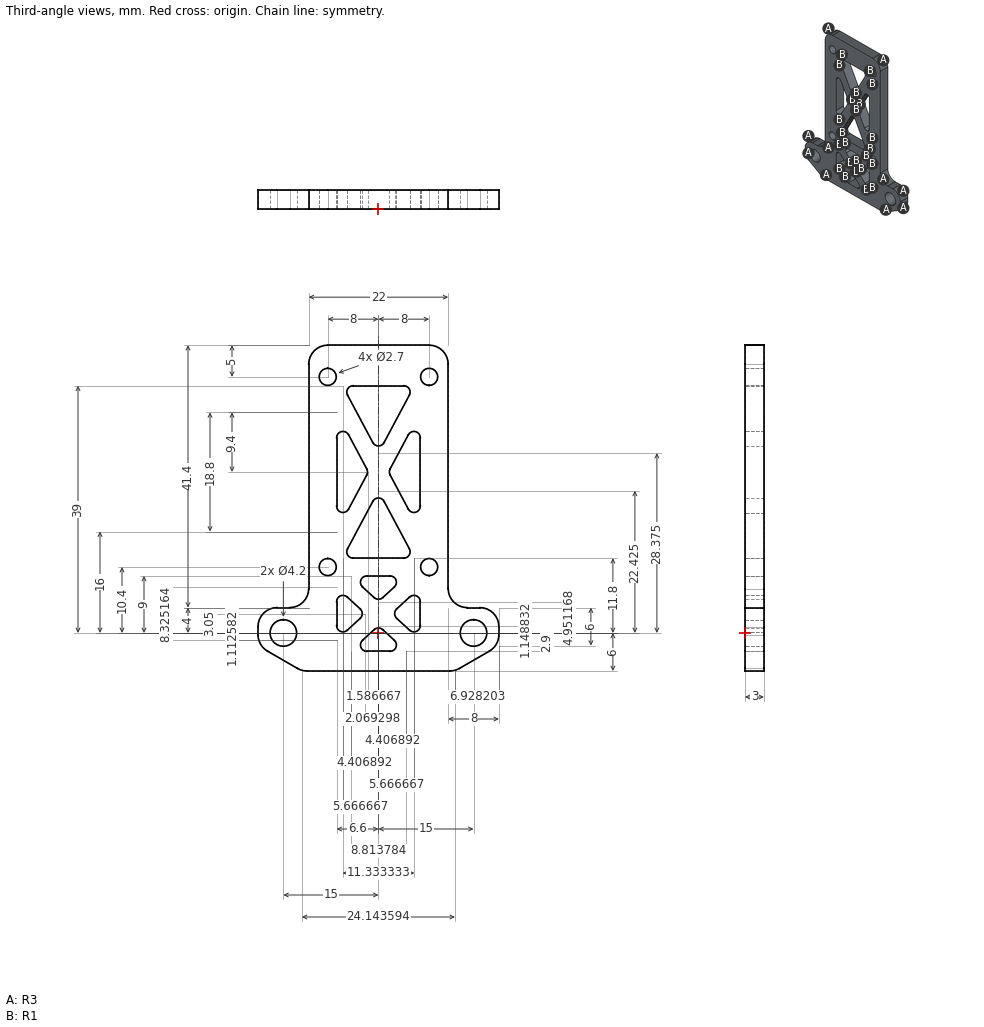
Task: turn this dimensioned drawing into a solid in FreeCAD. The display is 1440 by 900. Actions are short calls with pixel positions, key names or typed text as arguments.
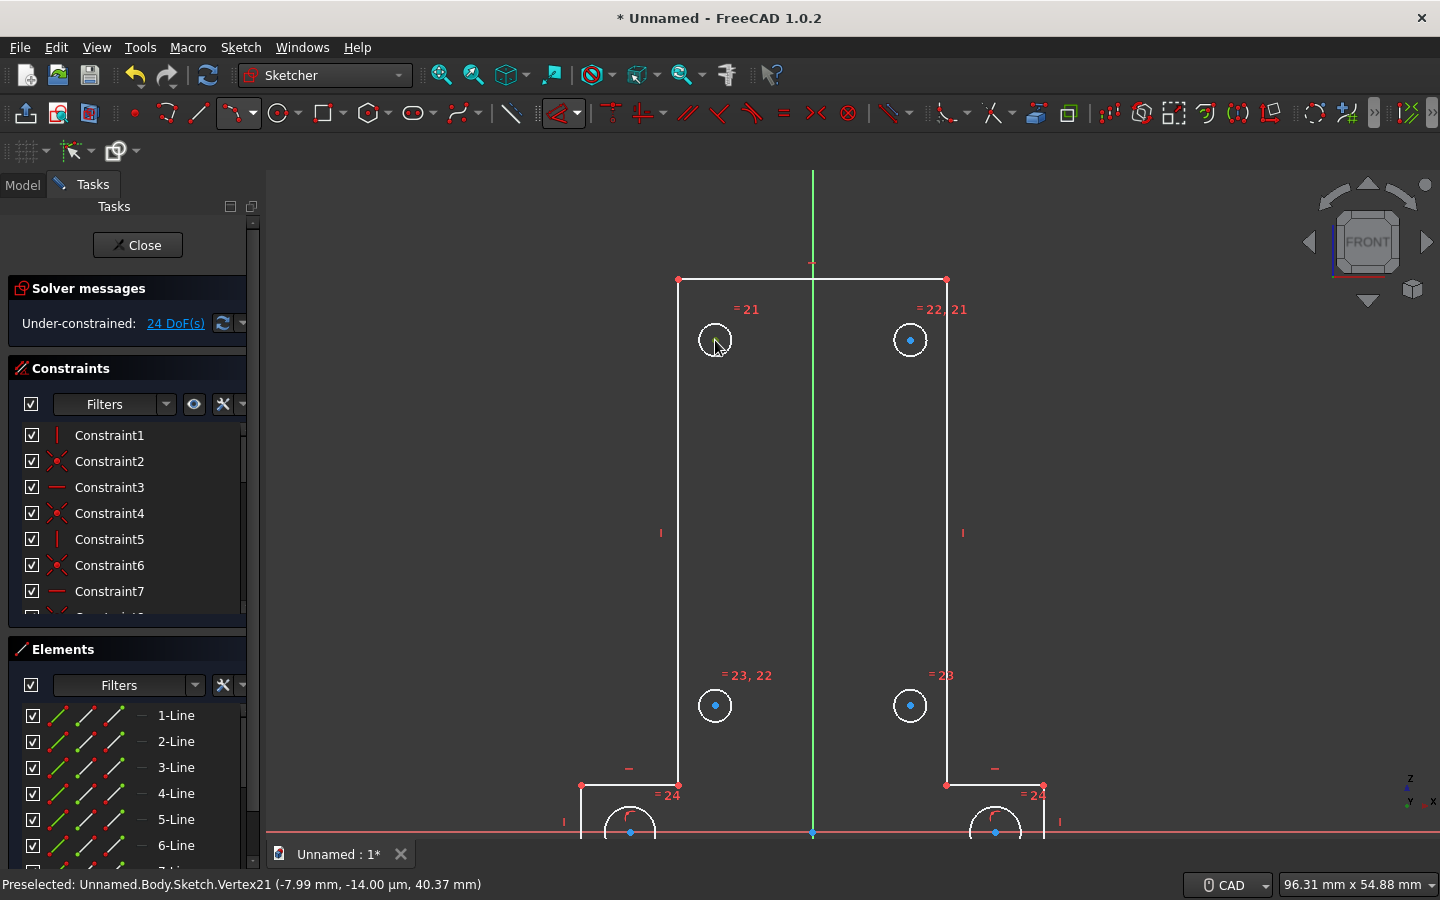
click(910, 340)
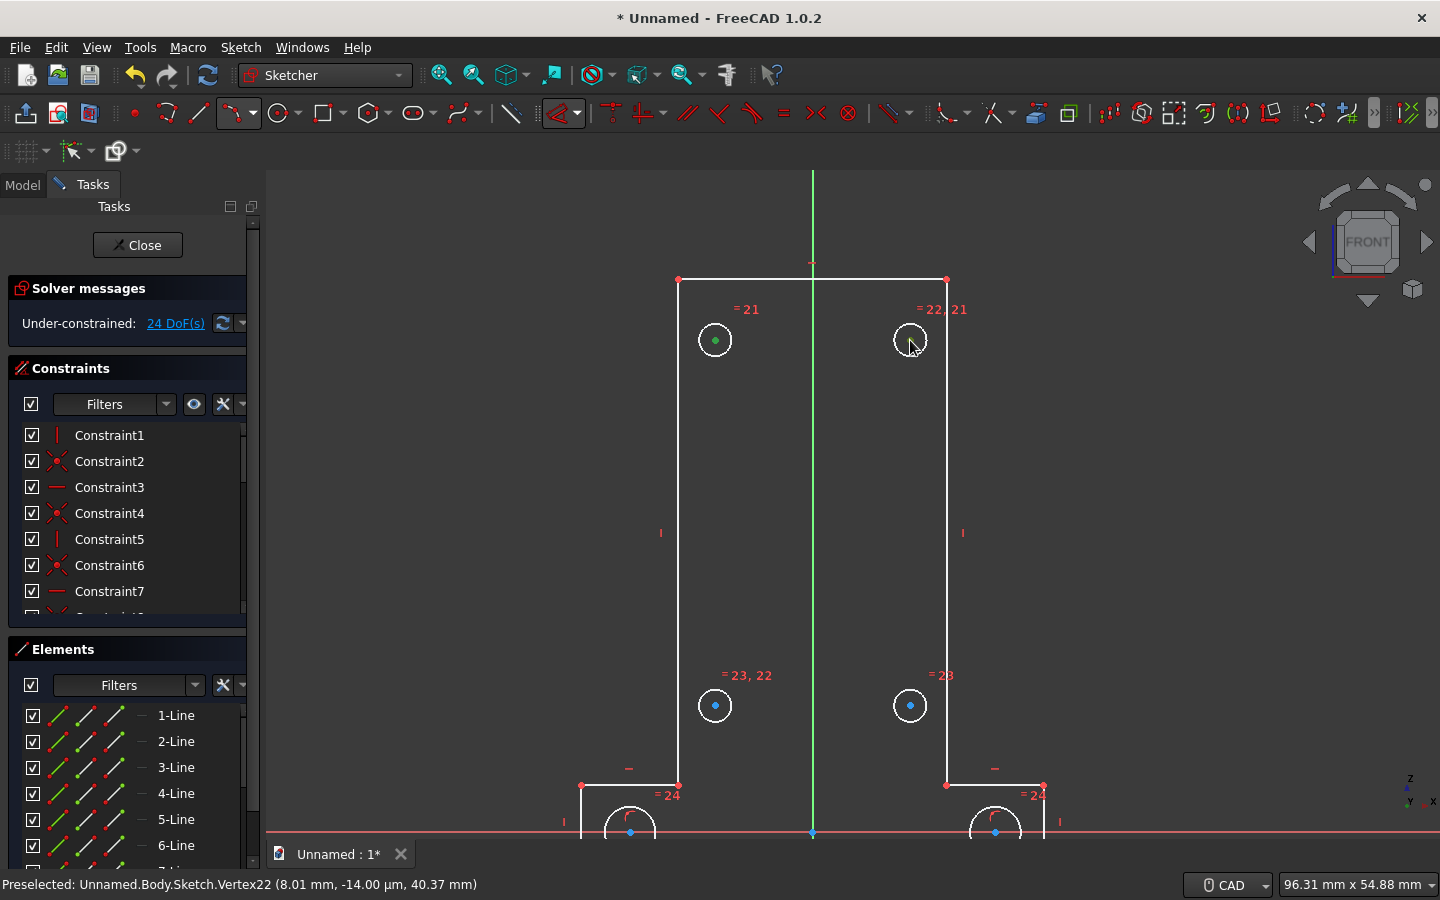
click(666, 114)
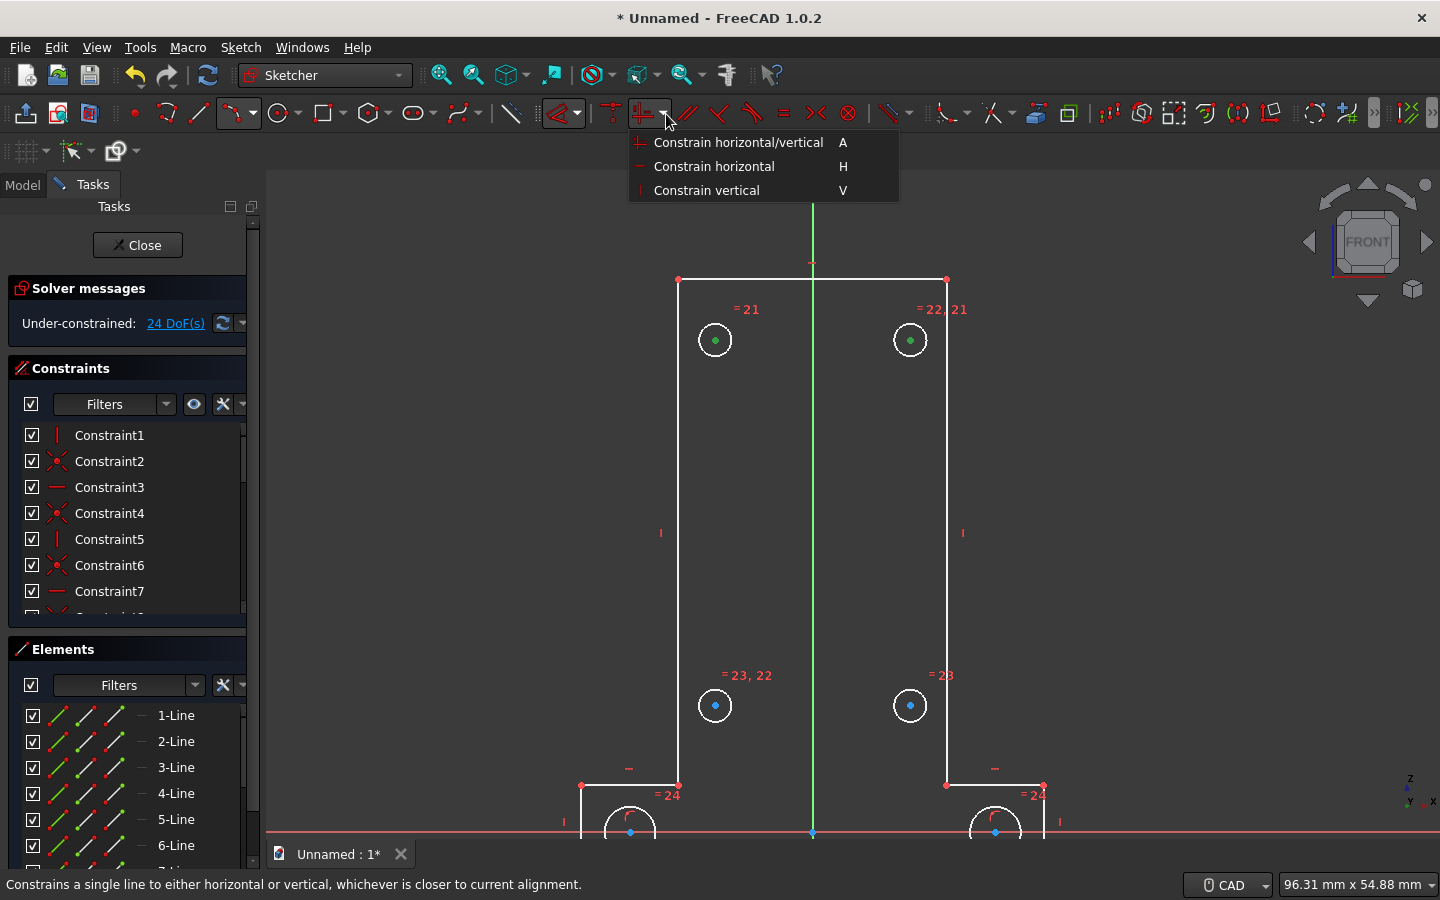
click(764, 166)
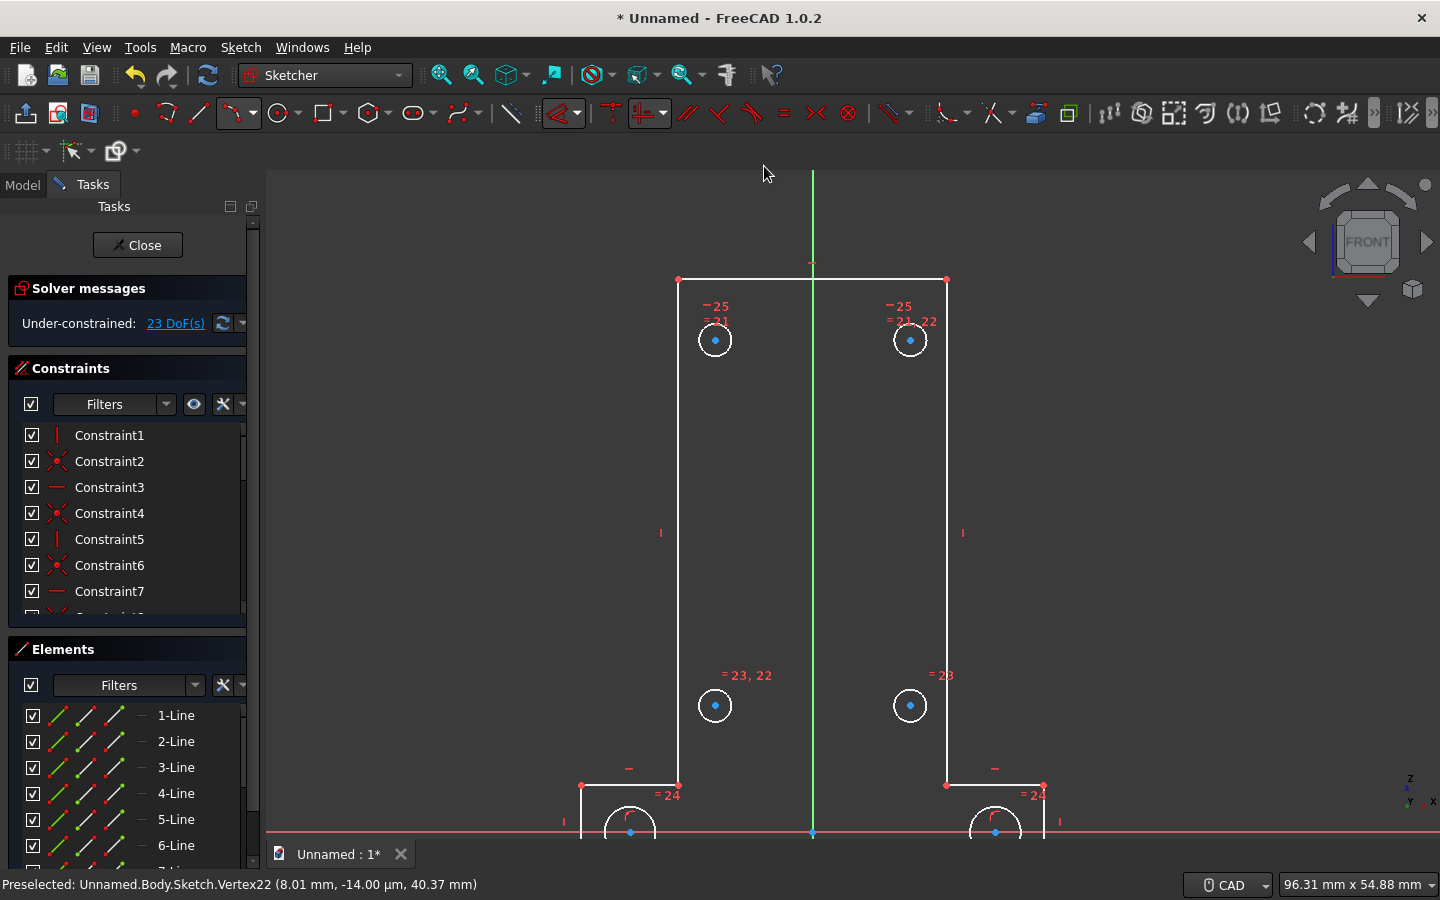
click(715, 706)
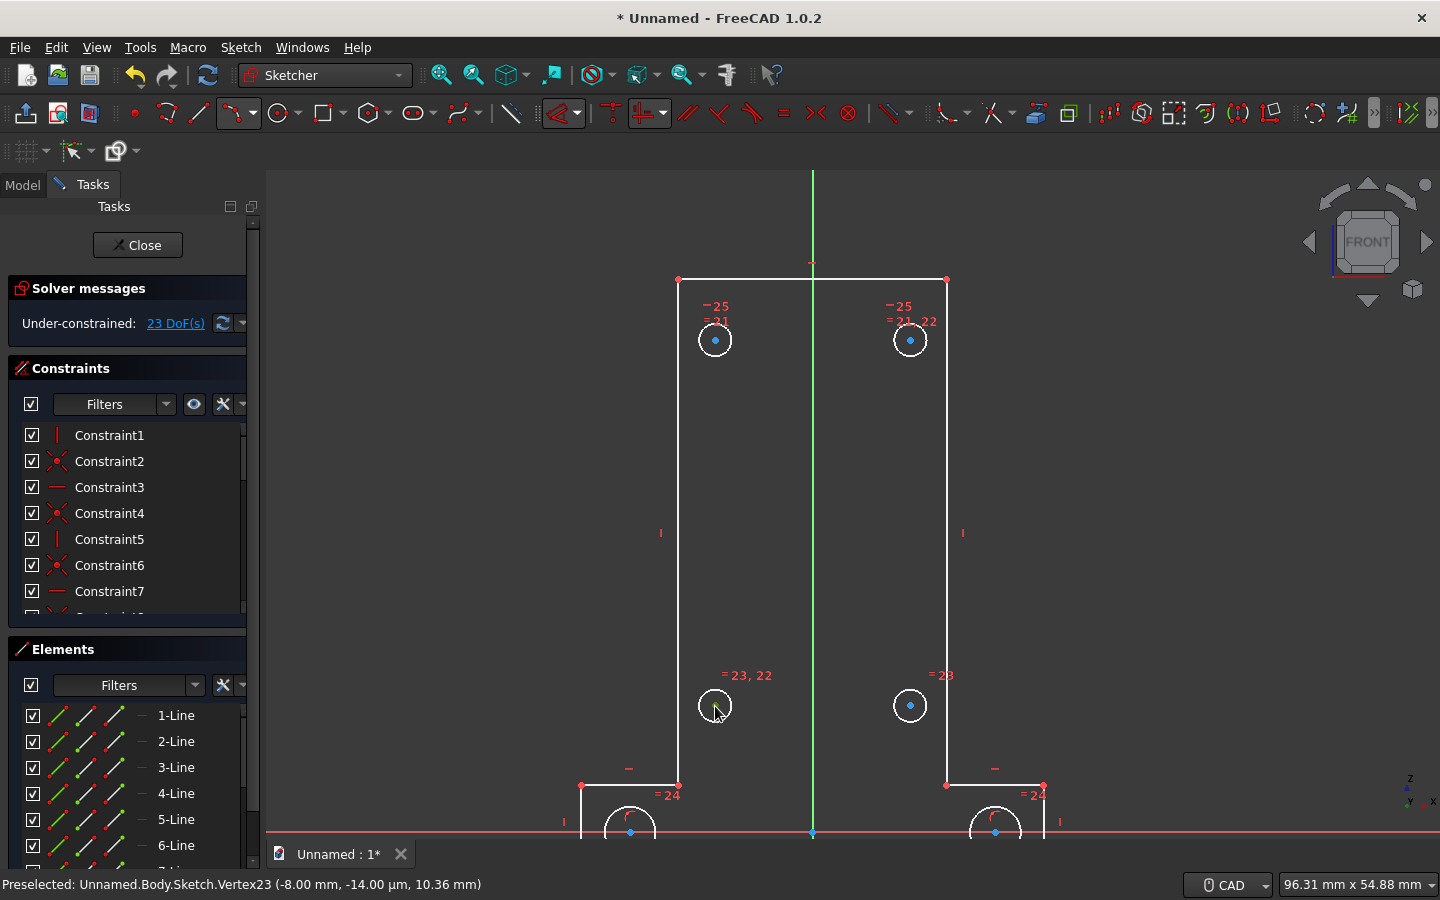
click(910, 706)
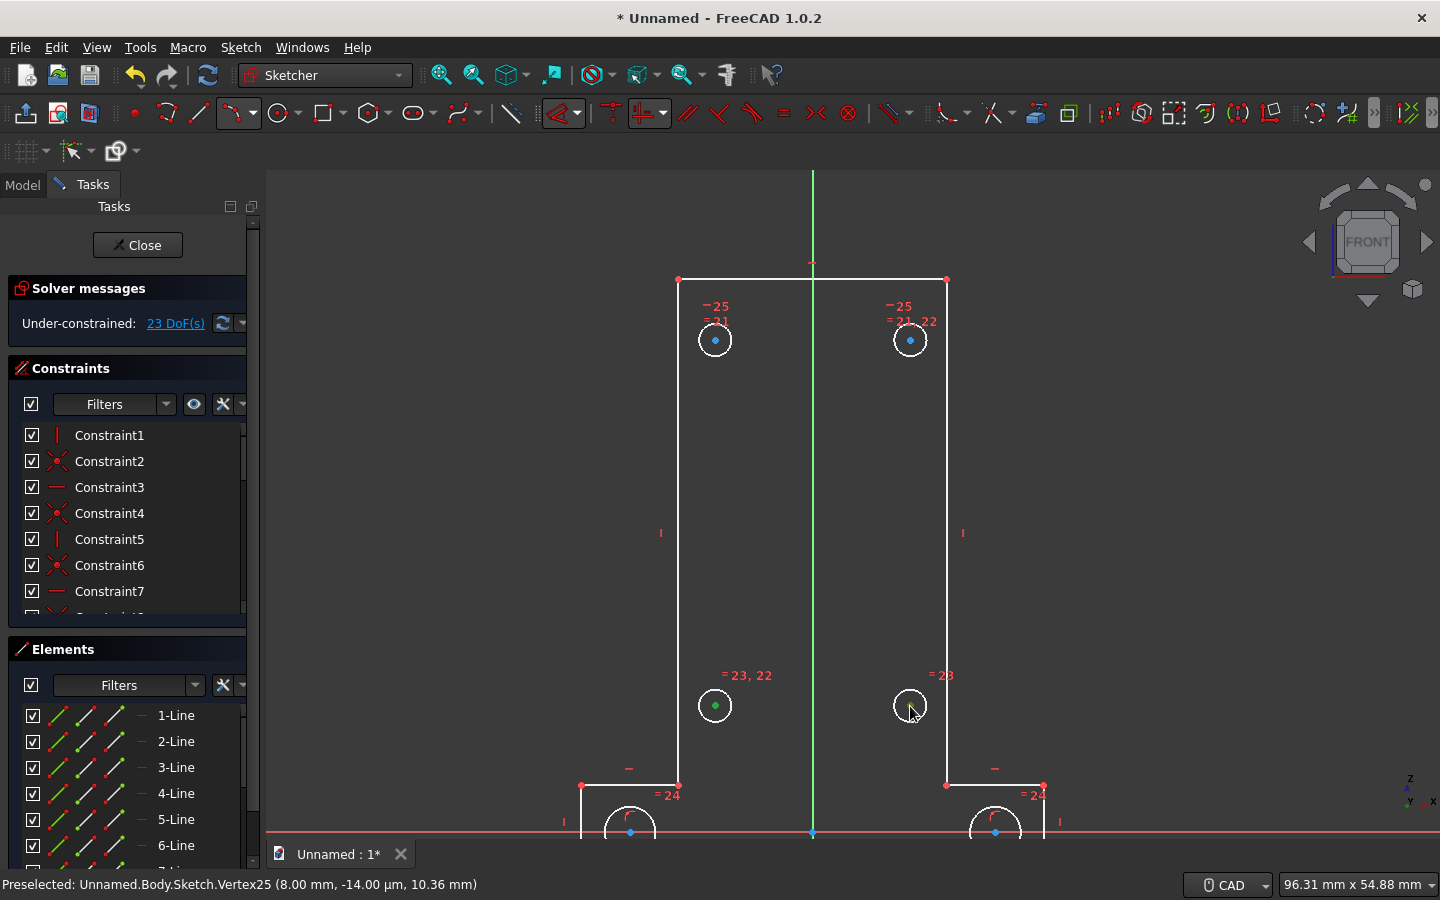
key(h)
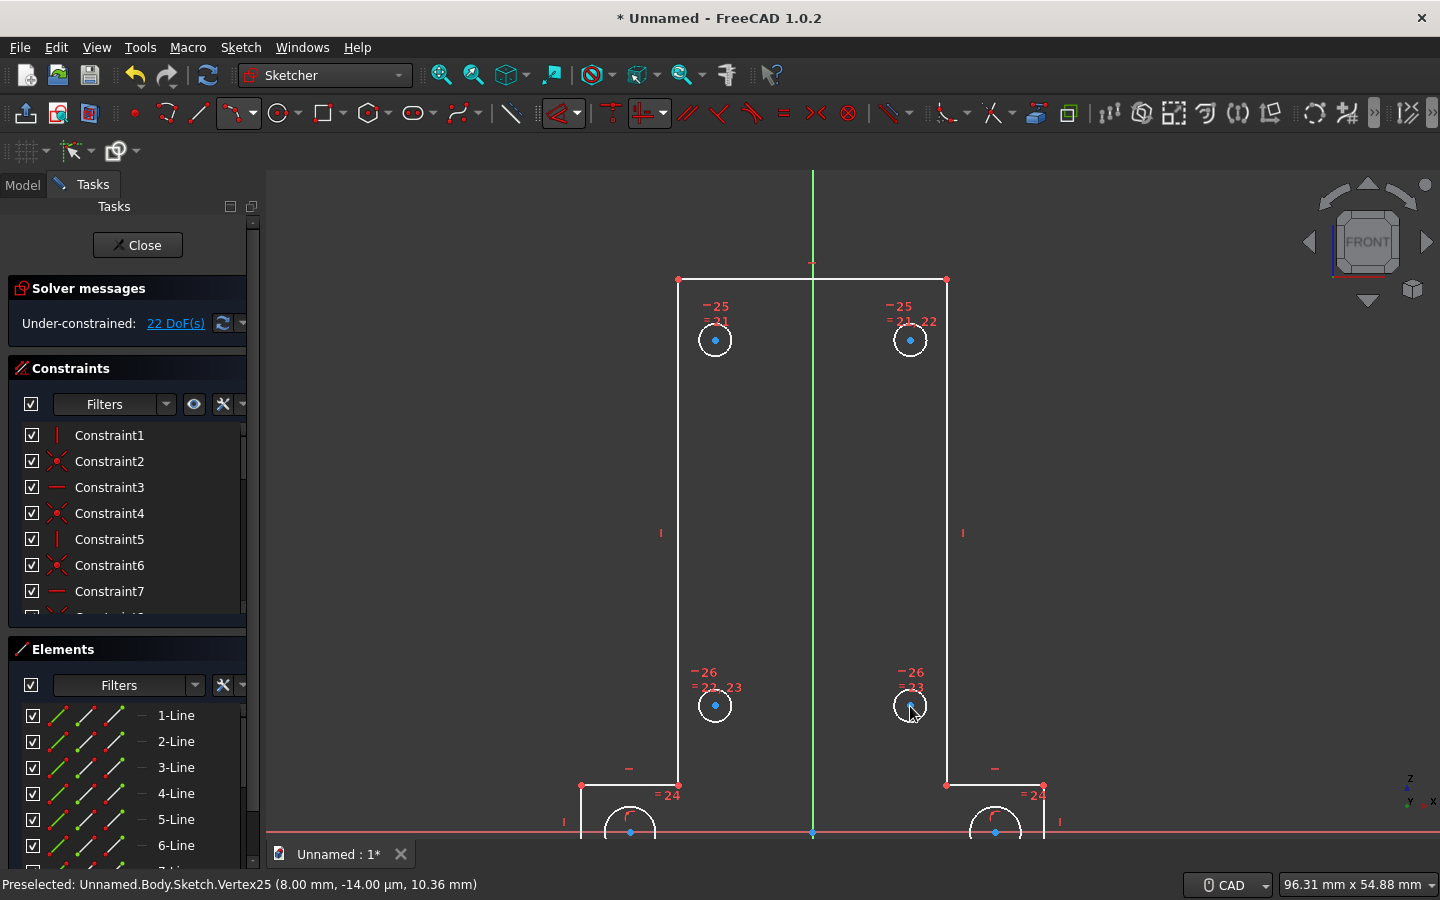
click(678, 785)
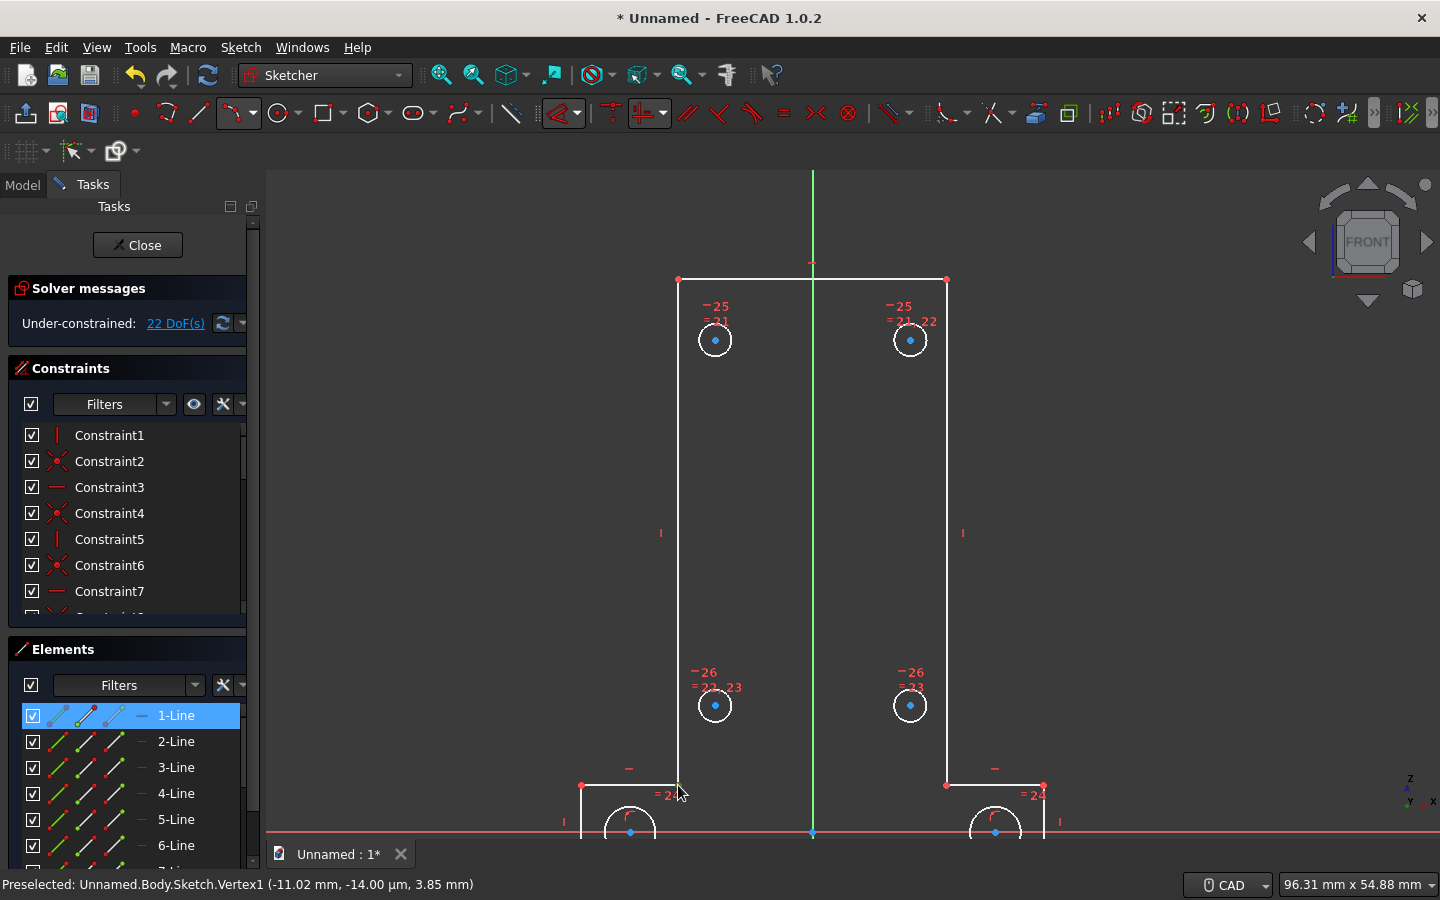
click(947, 785)